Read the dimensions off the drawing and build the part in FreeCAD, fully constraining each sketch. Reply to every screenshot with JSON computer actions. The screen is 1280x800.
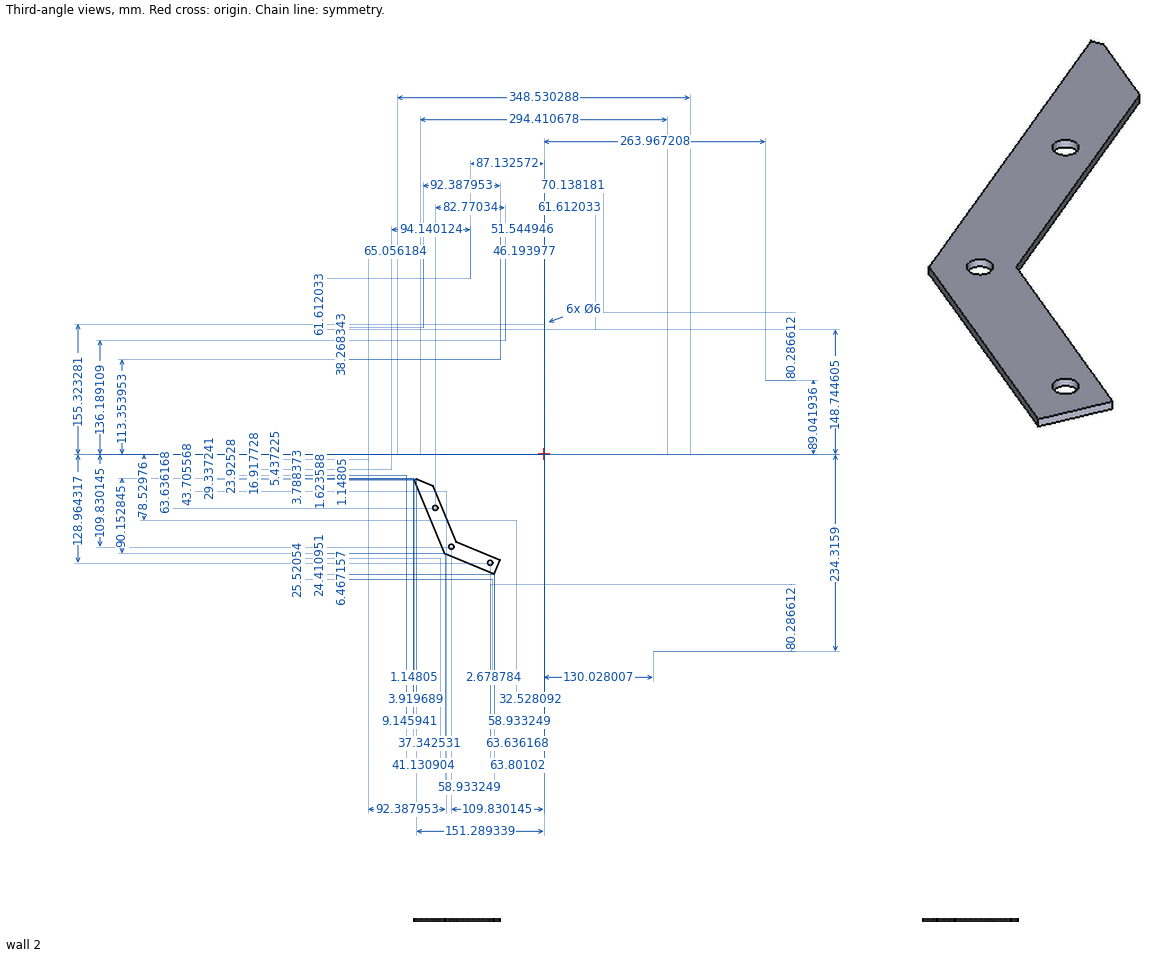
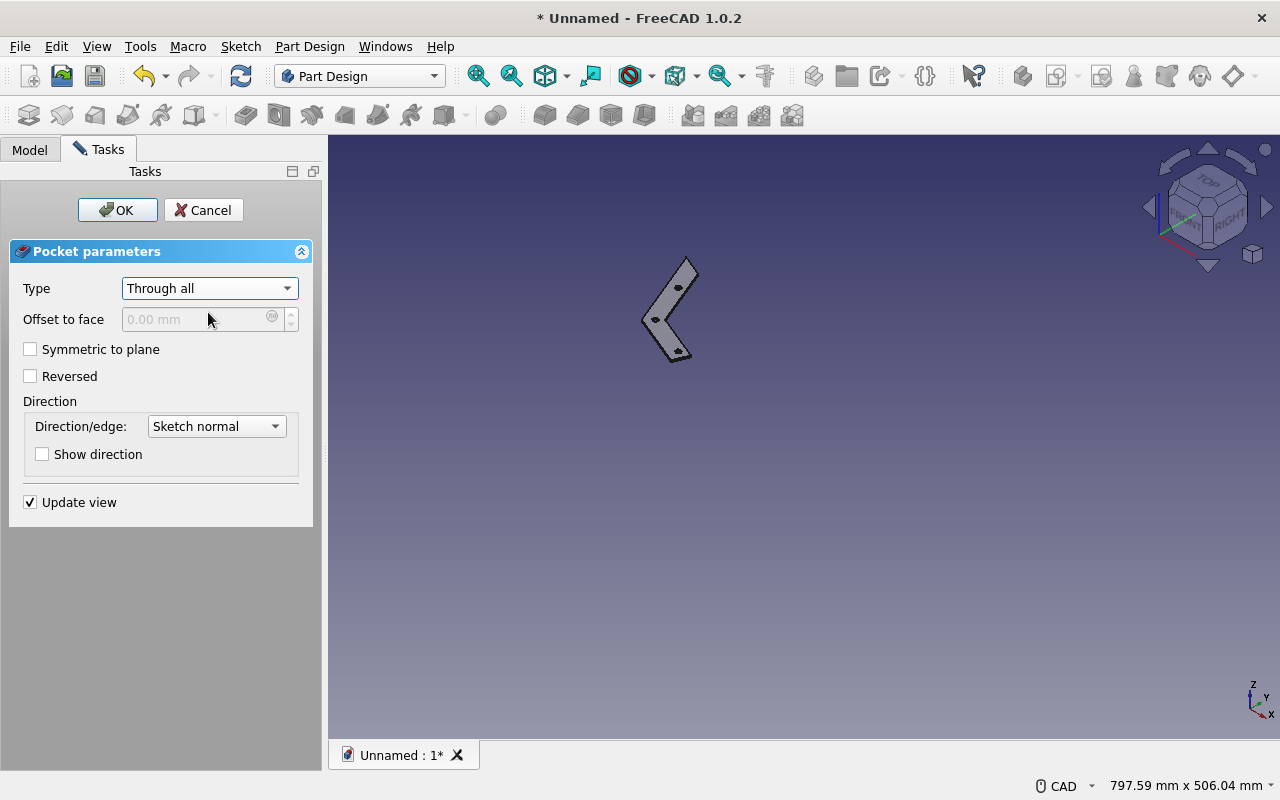
{"action": "left_click", "coordinate": [118, 210]}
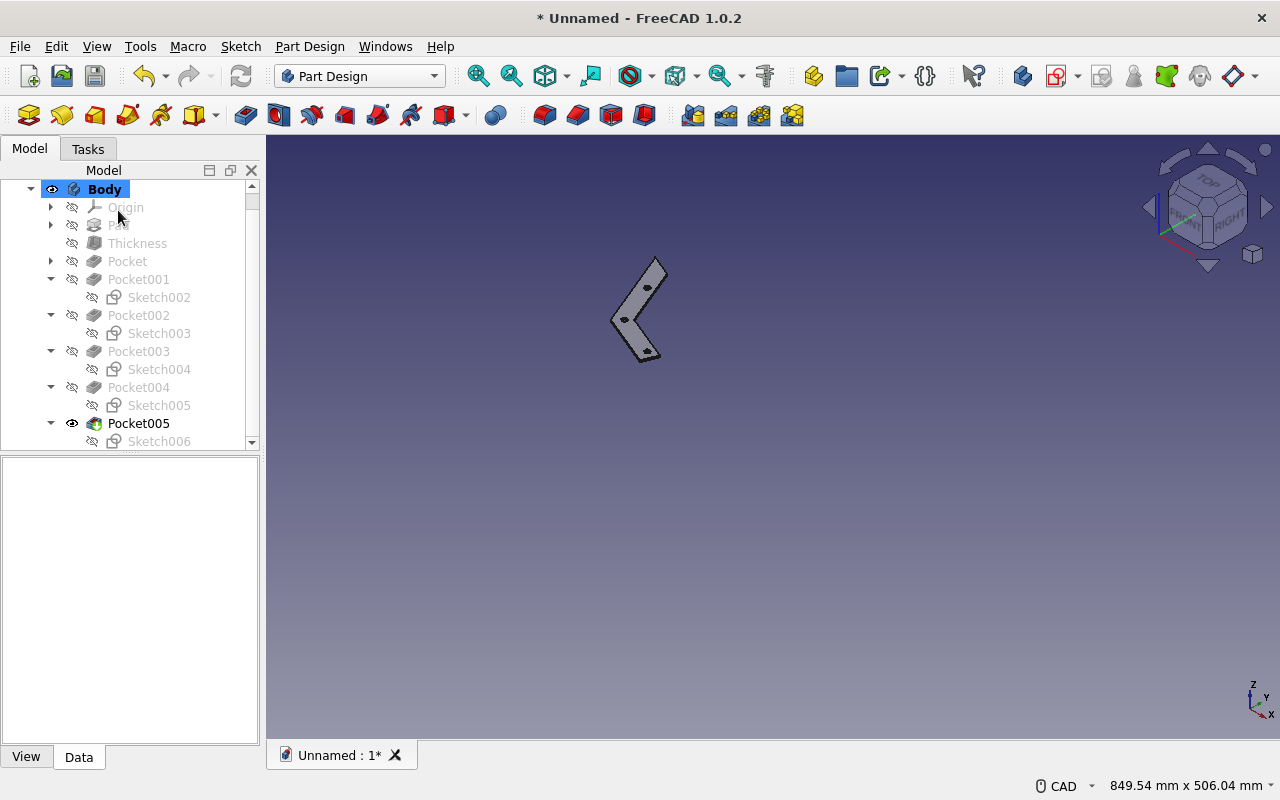
{"action": "left_click", "coordinate": [479, 76]}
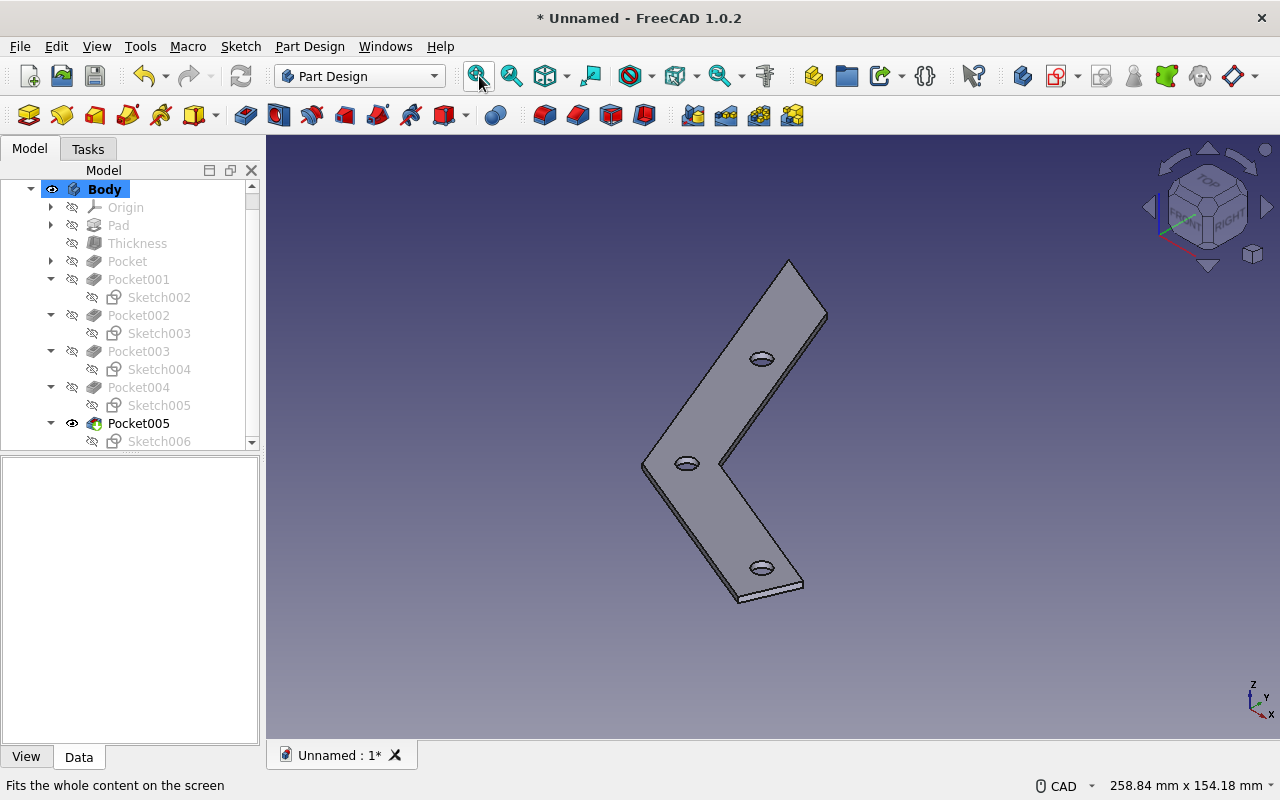
{"action": "left_click", "coordinate": [782, 333]}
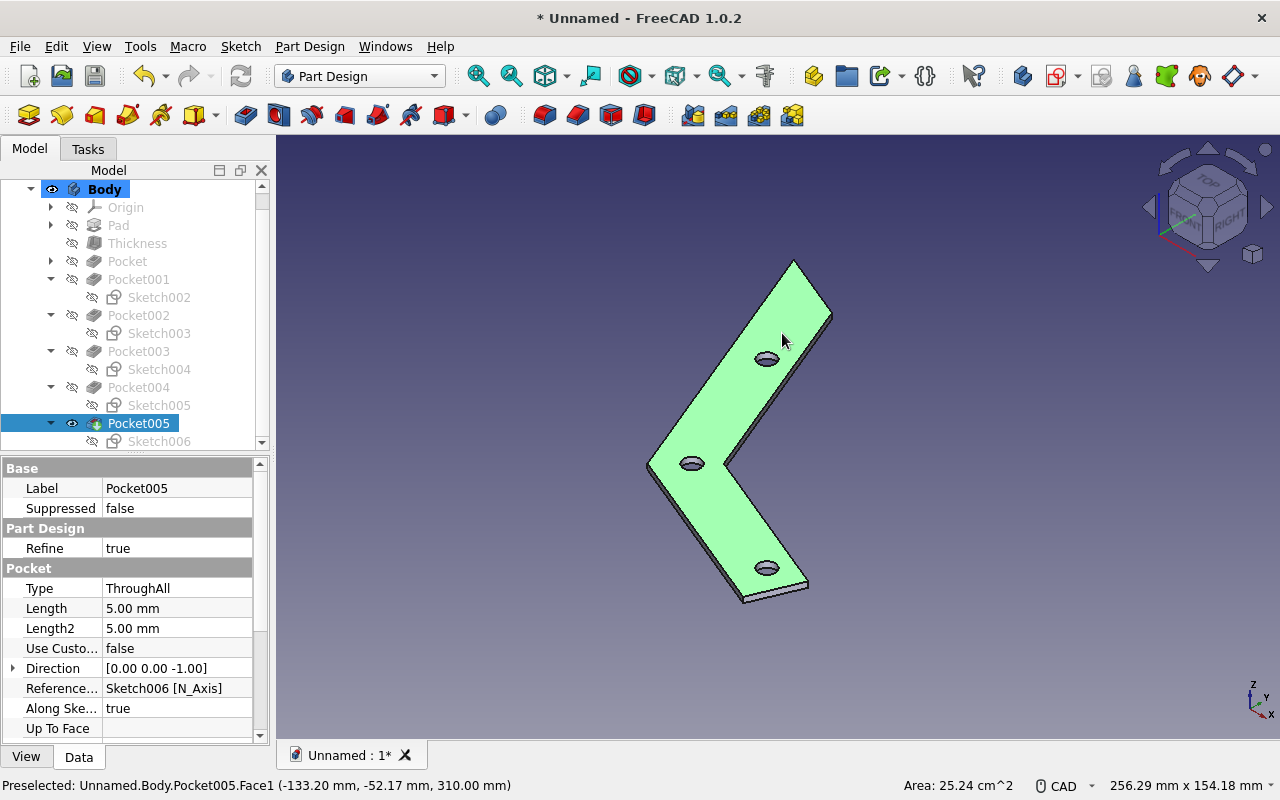
{"action": "left_click", "coordinate": [1056, 76]}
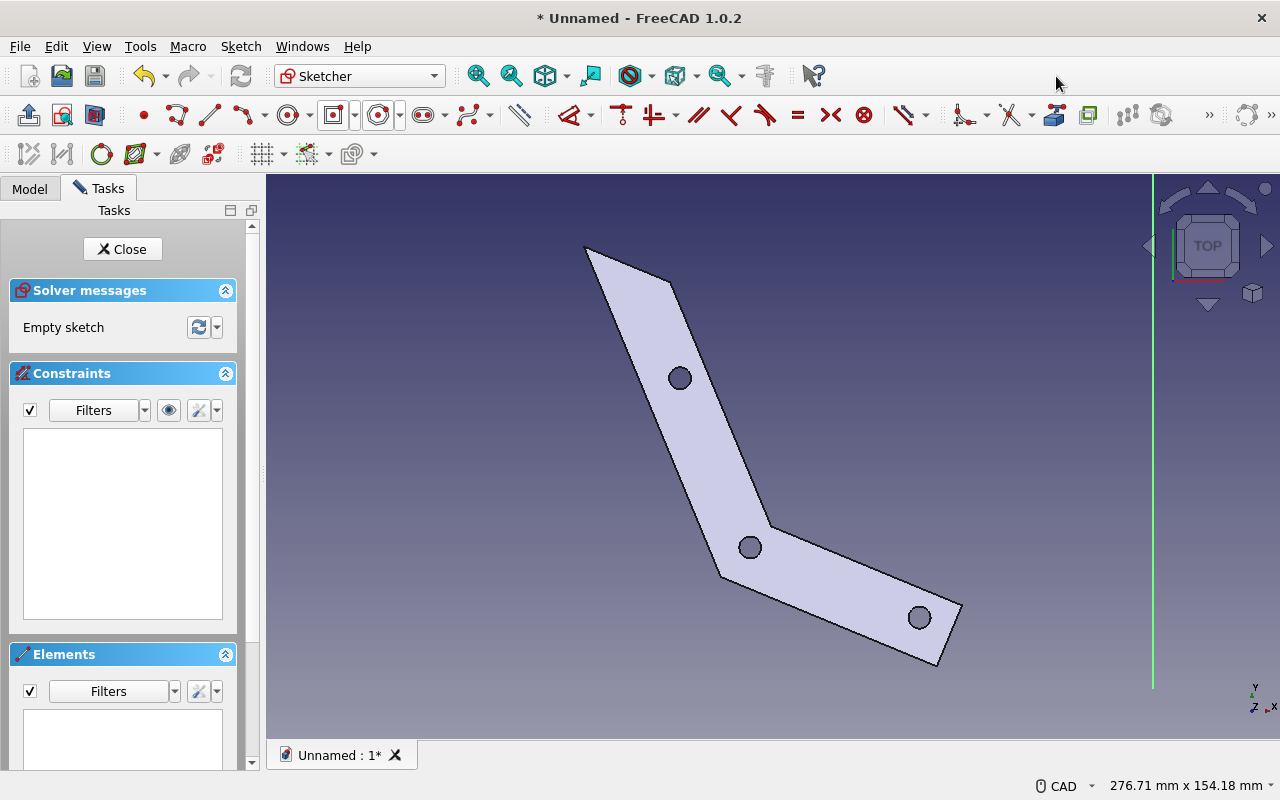
{"action": "scroll", "coordinate": [585, 241], "scroll_direction": "up", "scroll_amount": 15}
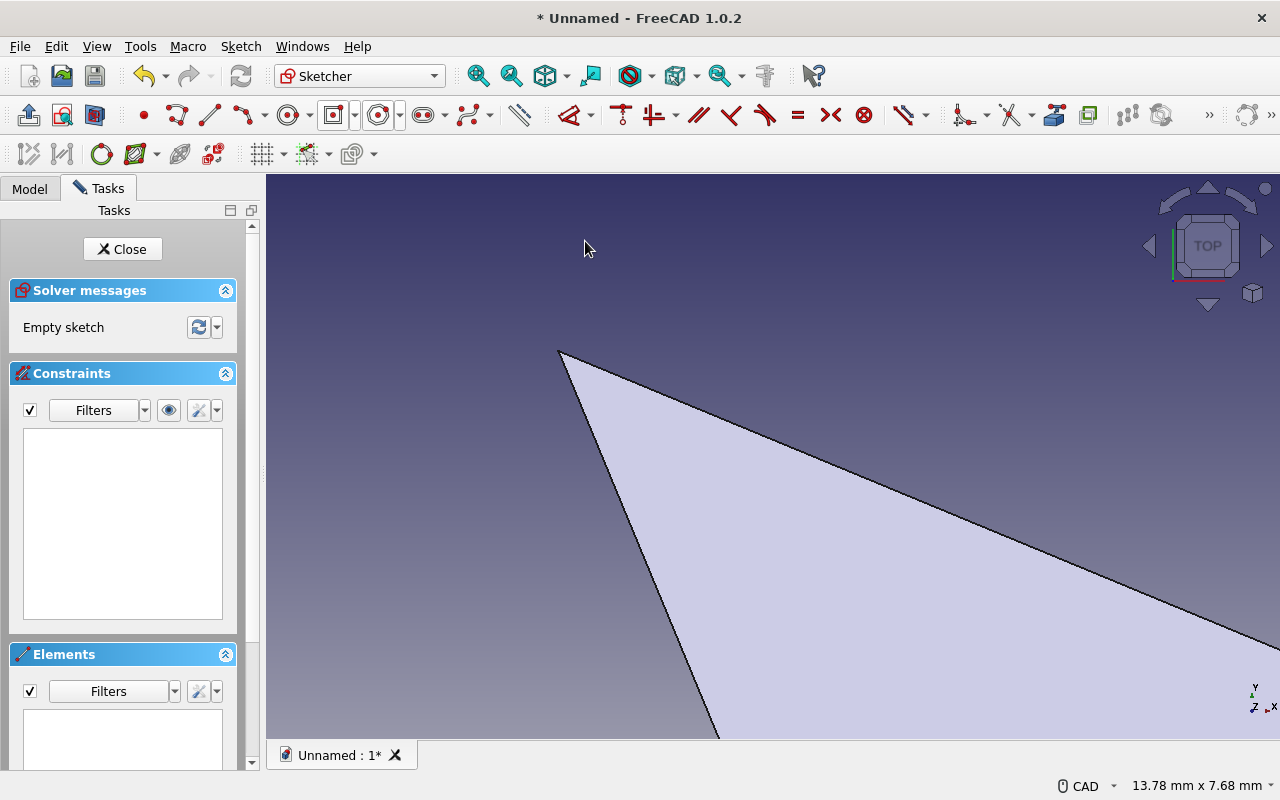
{"action": "scroll", "coordinate": [700, 449], "scroll_direction": "up", "scroll_amount": 3}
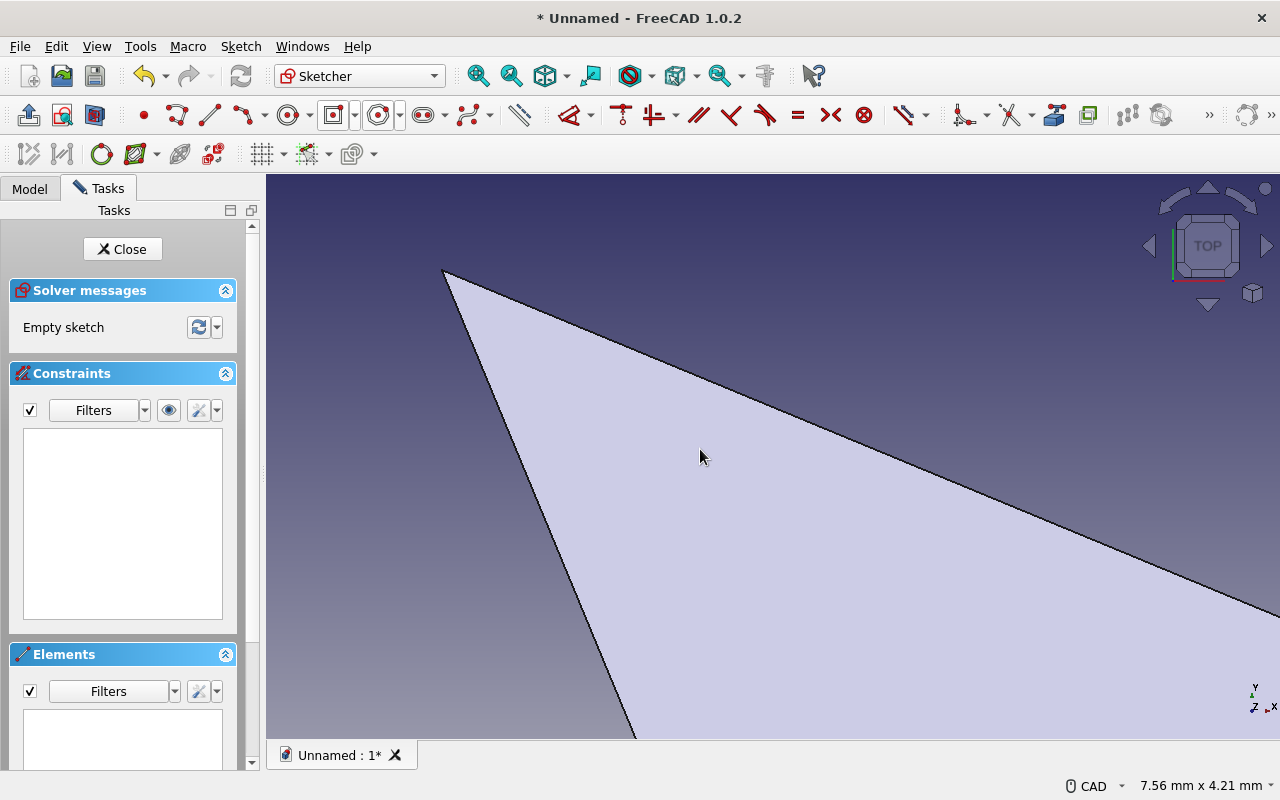
{"action": "left_click", "coordinate": [177, 116]}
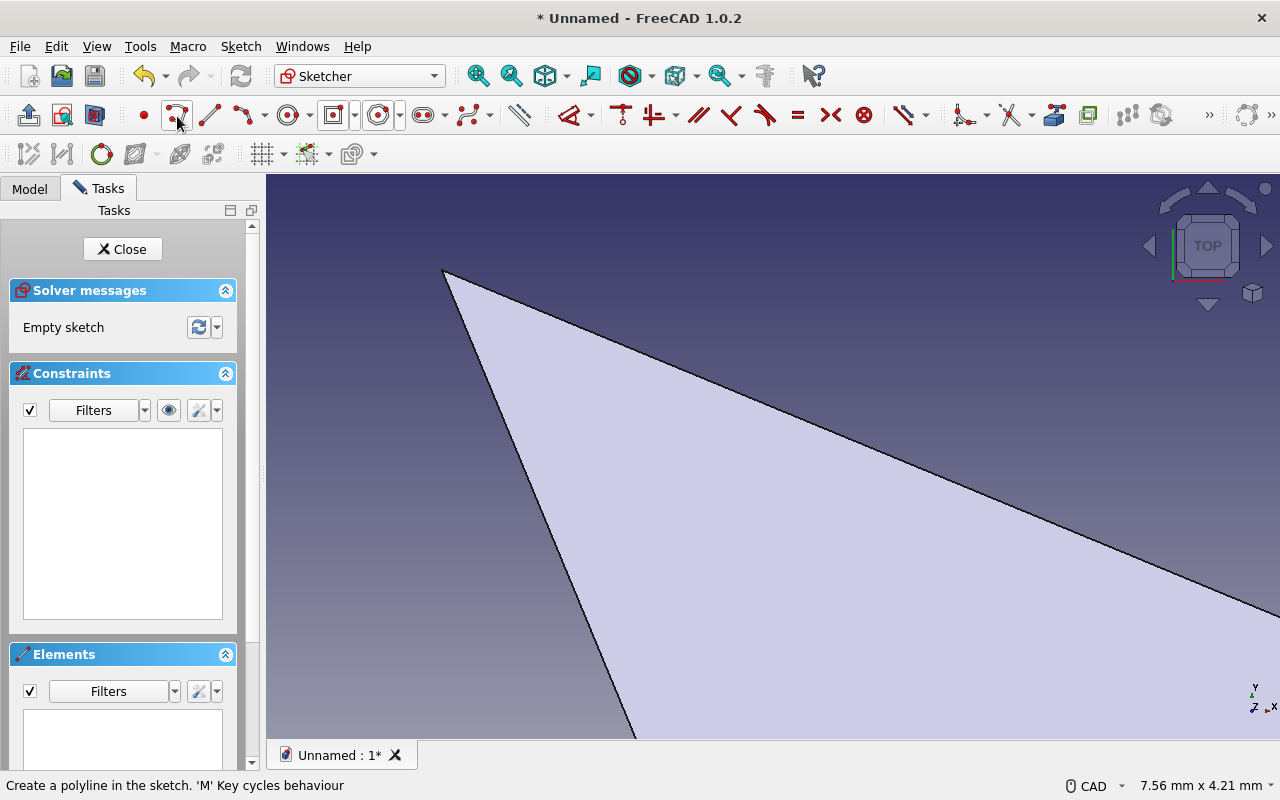
{"action": "left_click", "coordinate": [967, 488]}
{"action": "left_click", "coordinate": [442, 270]}
{"action": "left_click", "coordinate": [596, 642]}
{"action": "left_click", "coordinate": [967, 489]}
{"action": "key", "text": "Escape"}
{"action": "key", "text": "Escape"}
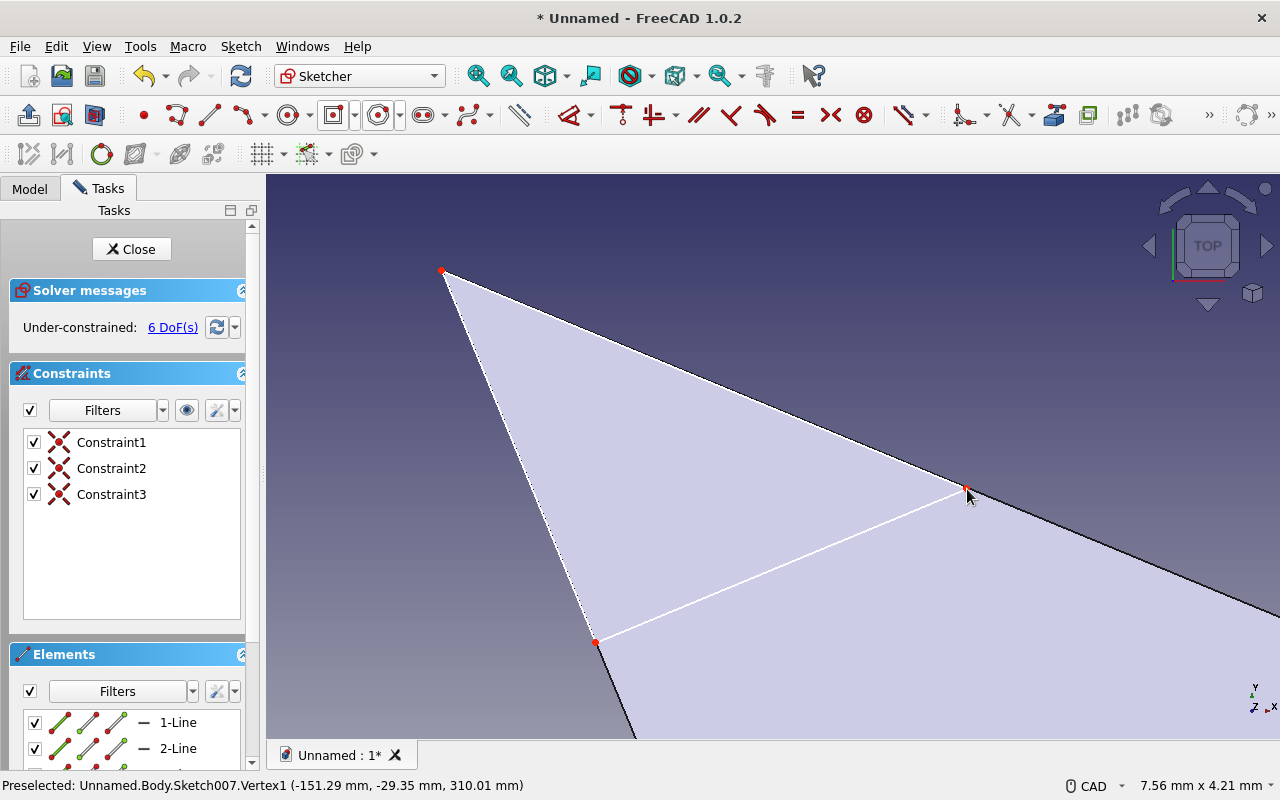
{"action": "left_click", "coordinate": [568, 116]}